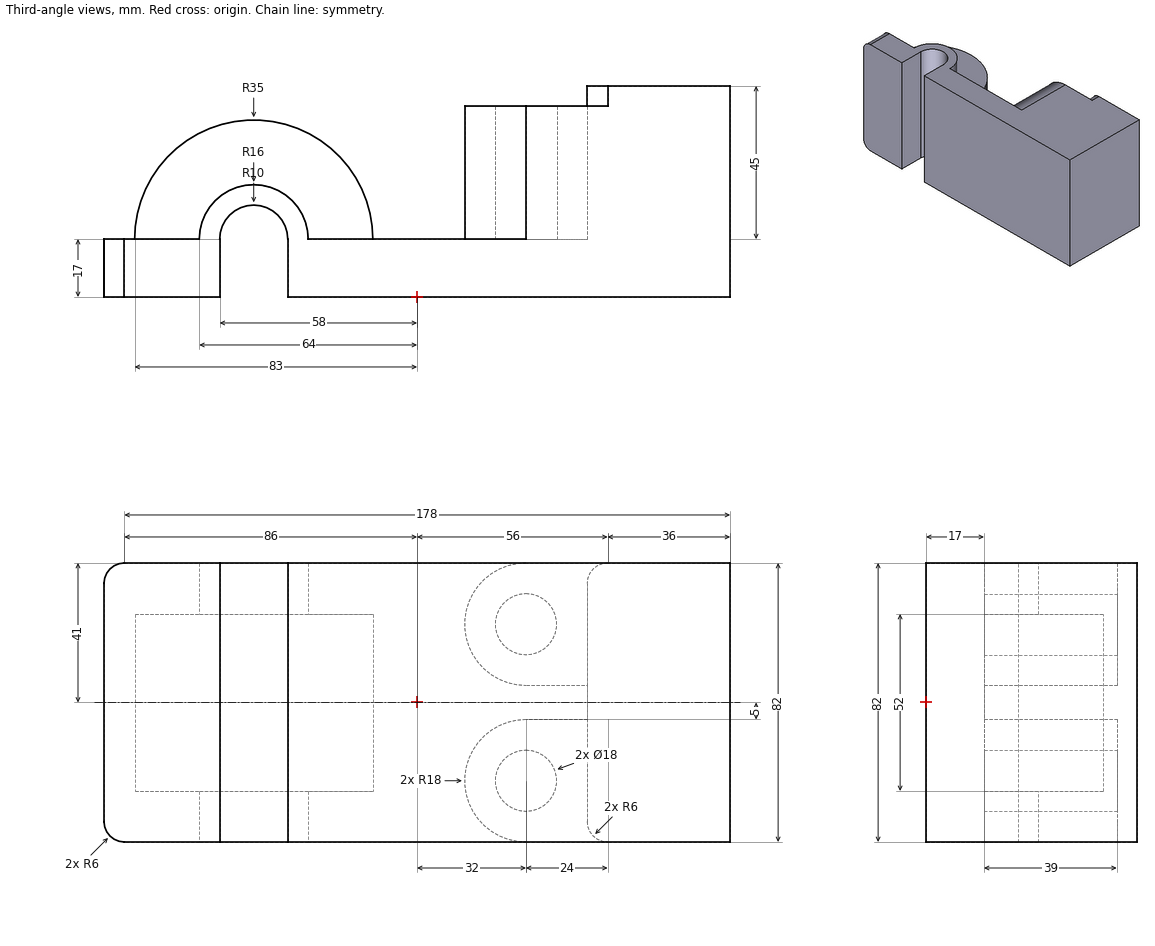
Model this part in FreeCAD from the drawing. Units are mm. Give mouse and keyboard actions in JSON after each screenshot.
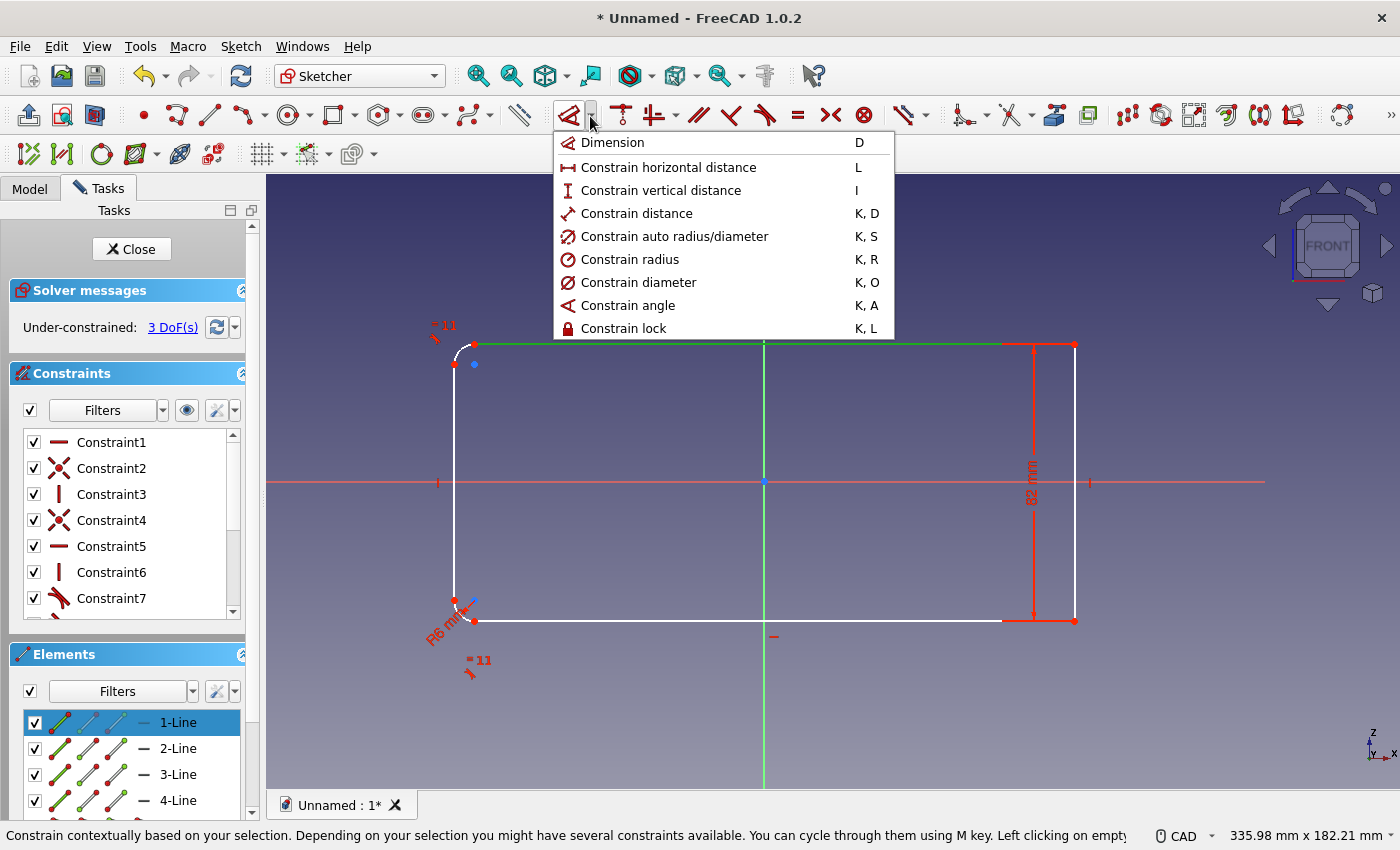
{"action": "left_click", "coordinate": [724, 168]}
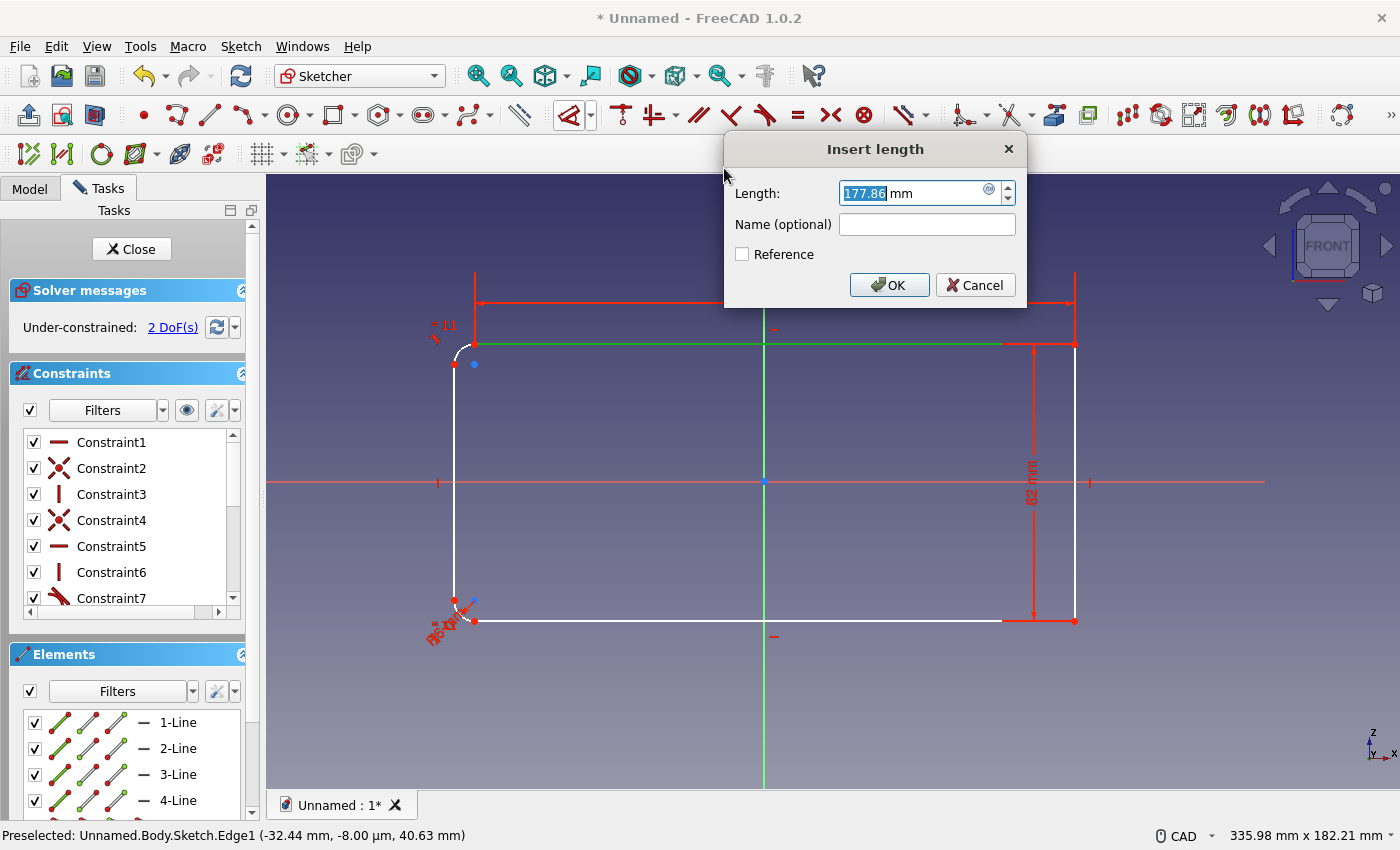
{"action": "type", "text": "178"}
{"action": "key", "text": "Return"}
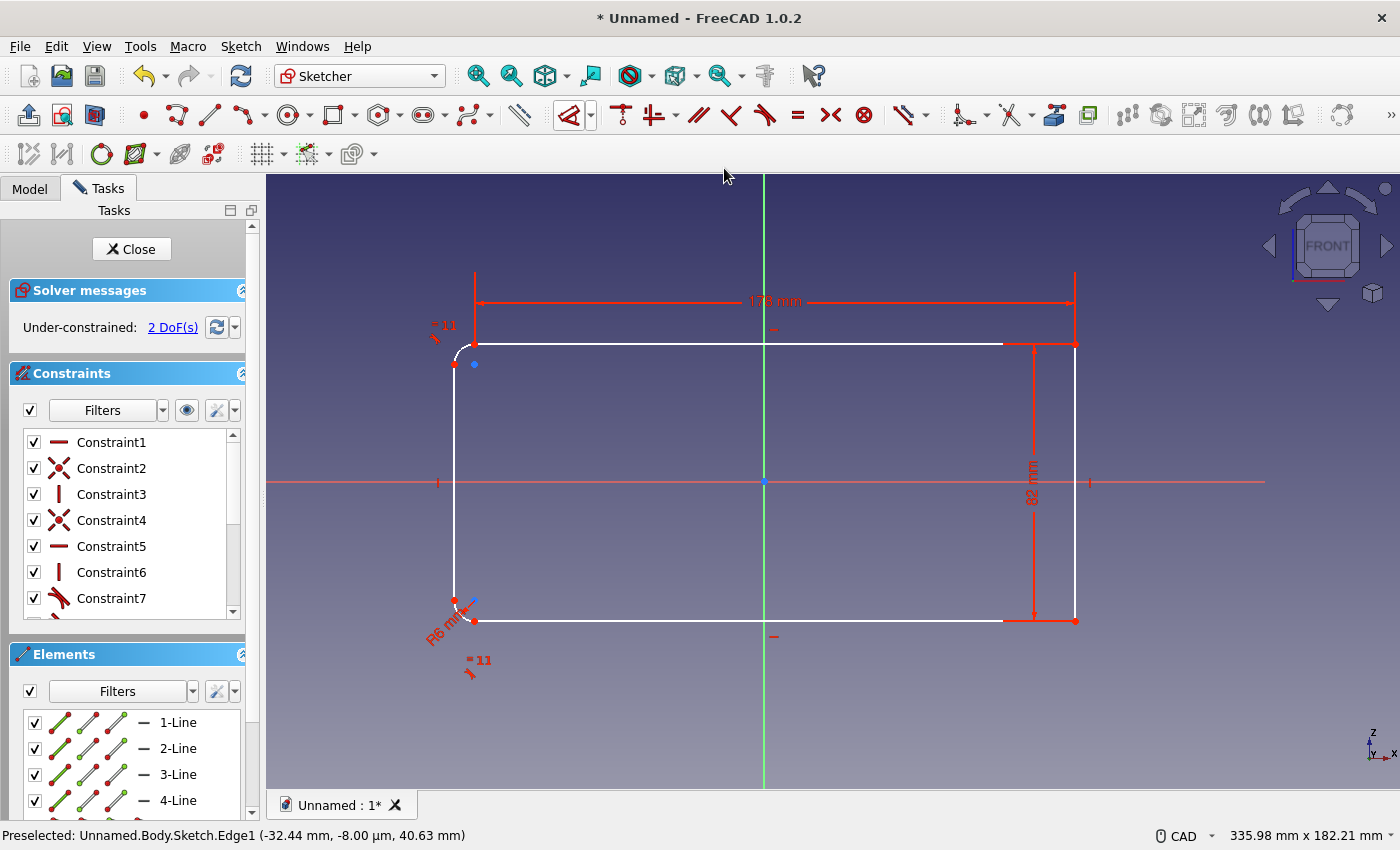
{"action": "left_click", "coordinate": [475, 344]}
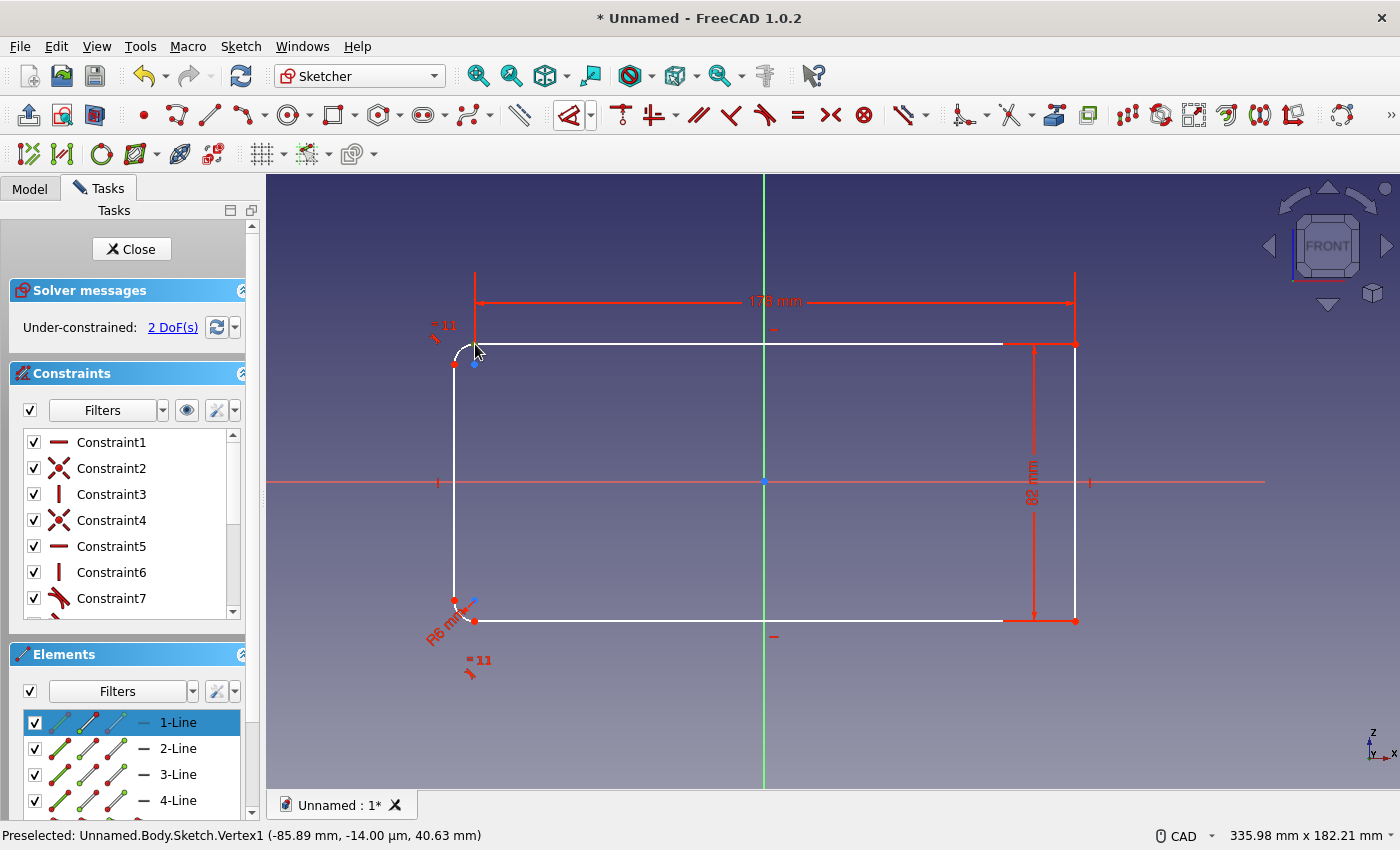
{"action": "left_click", "coordinate": [590, 116]}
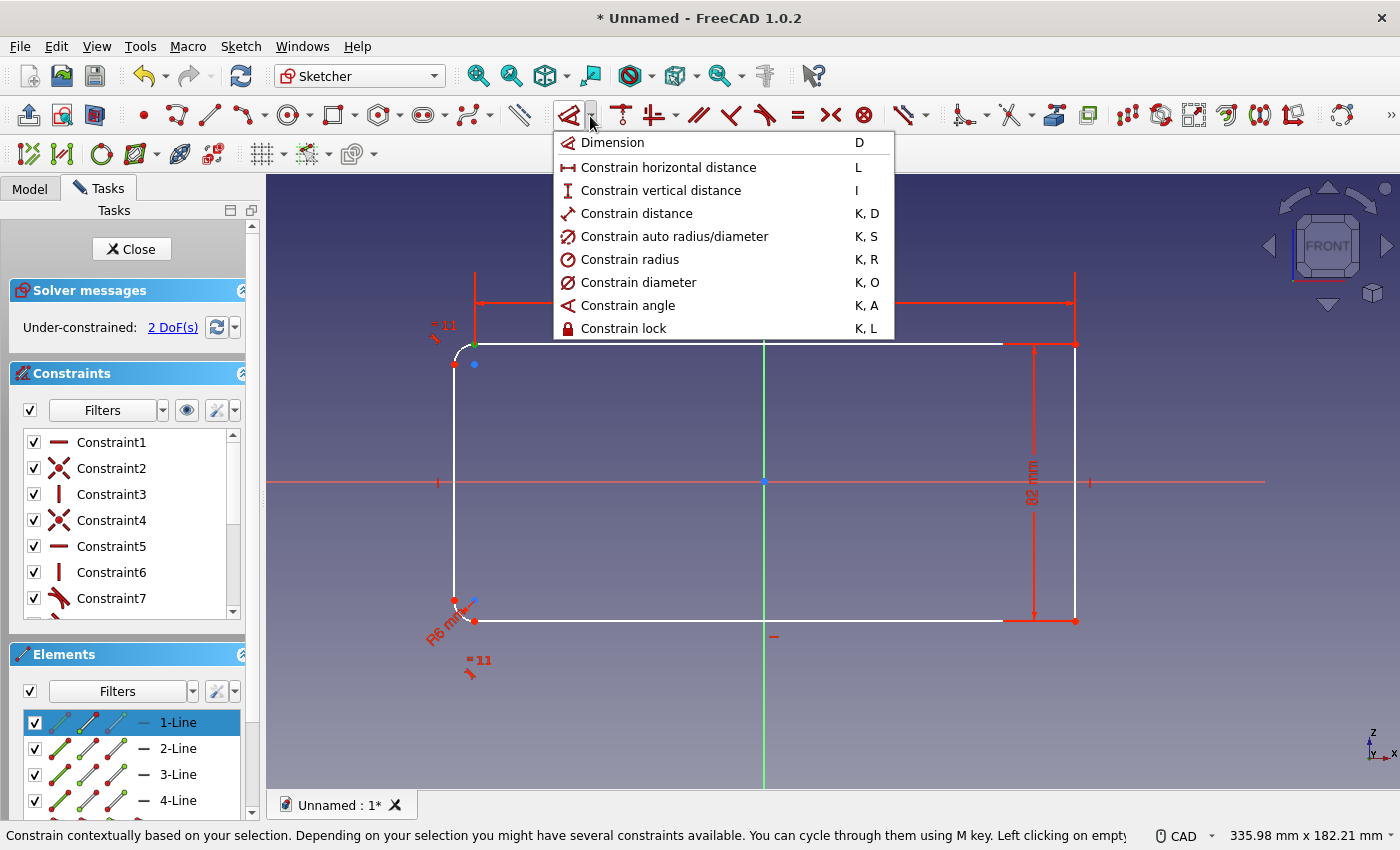
{"action": "left_click", "coordinate": [724, 168]}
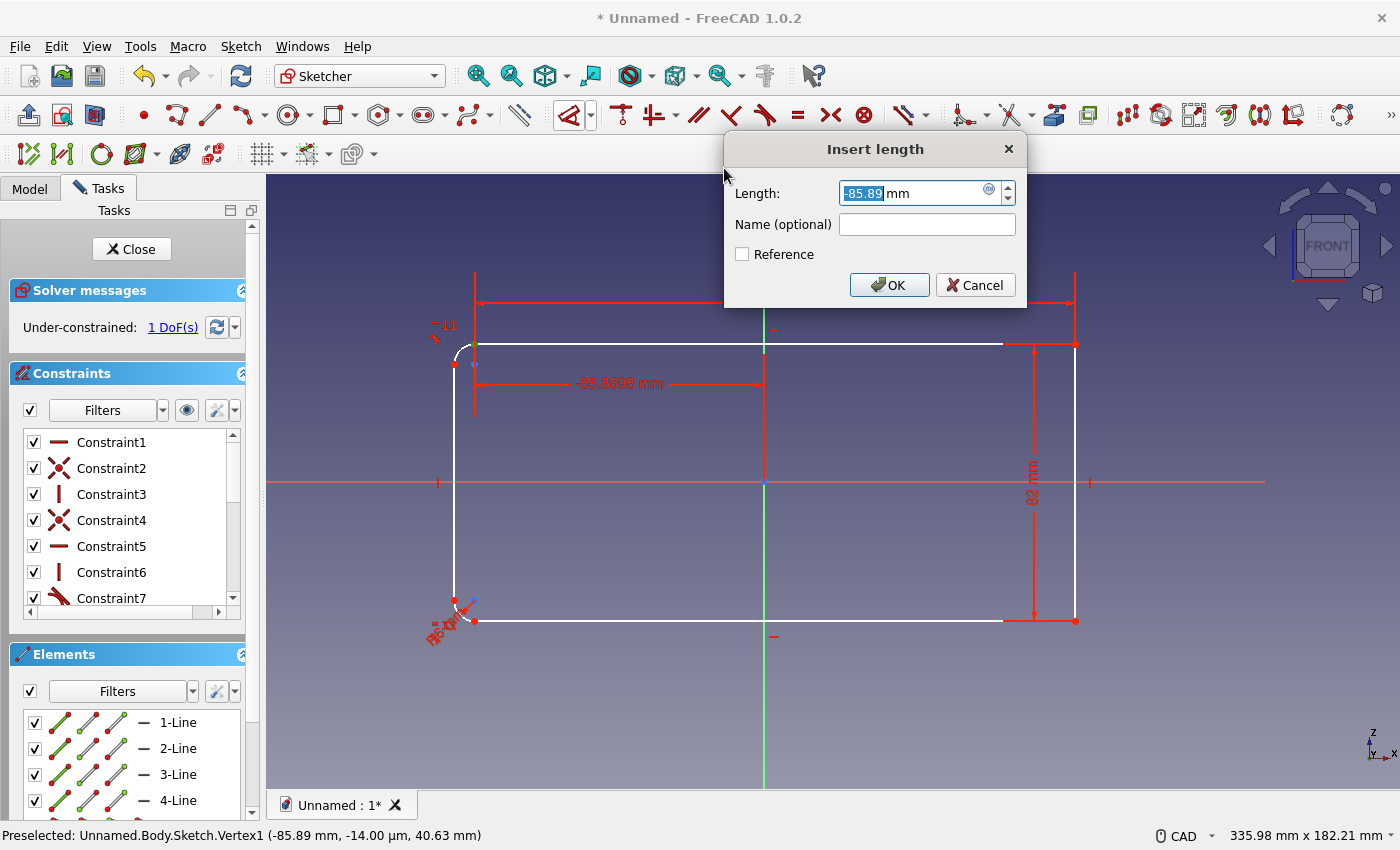
{"action": "type", "text": "-86"}
{"action": "key", "text": "Return"}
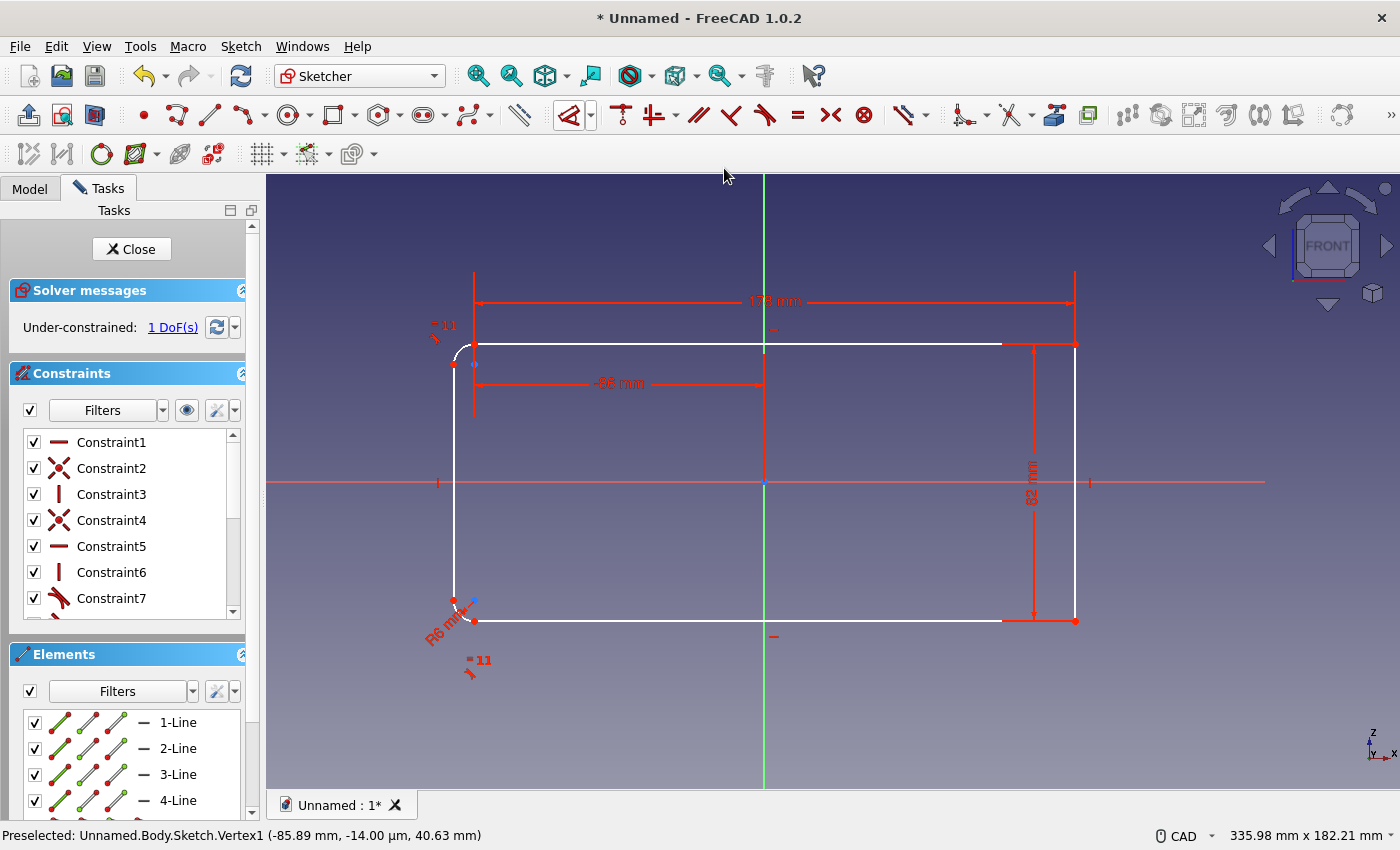
{"action": "left_click", "coordinate": [474, 344]}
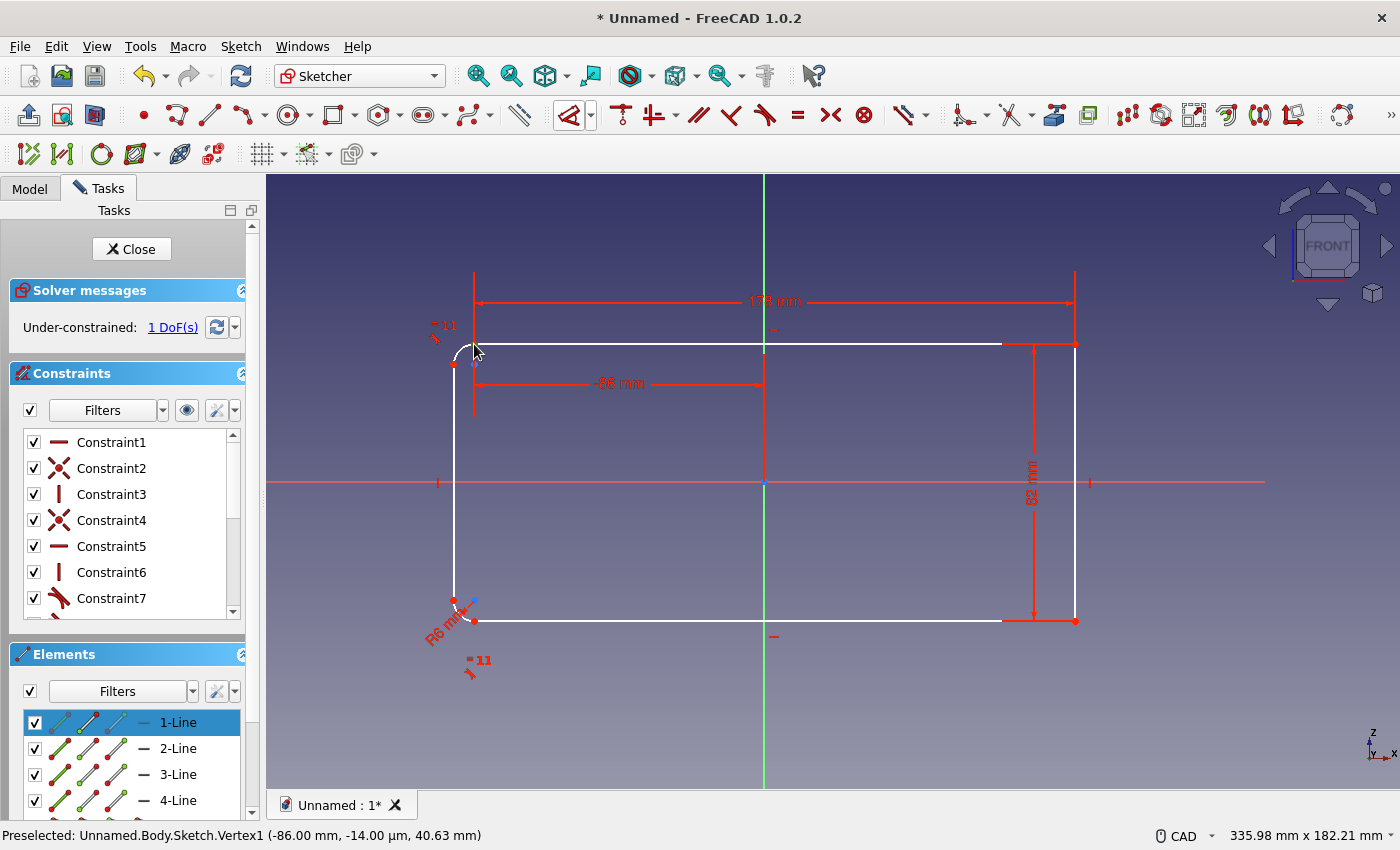
{"action": "left_click", "coordinate": [590, 116]}